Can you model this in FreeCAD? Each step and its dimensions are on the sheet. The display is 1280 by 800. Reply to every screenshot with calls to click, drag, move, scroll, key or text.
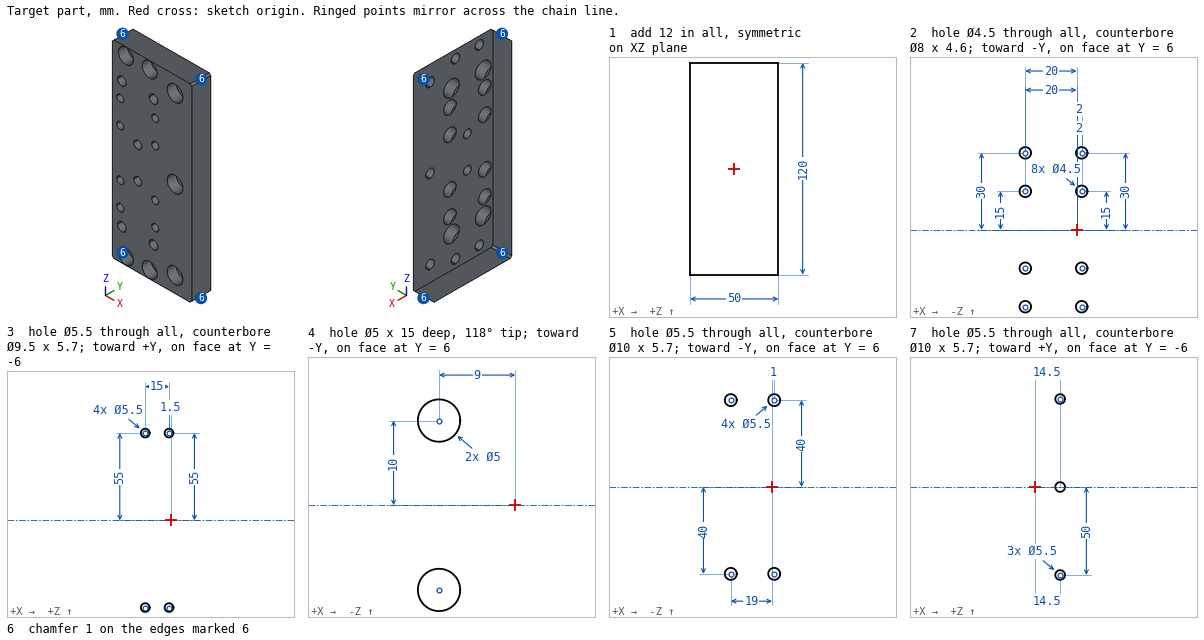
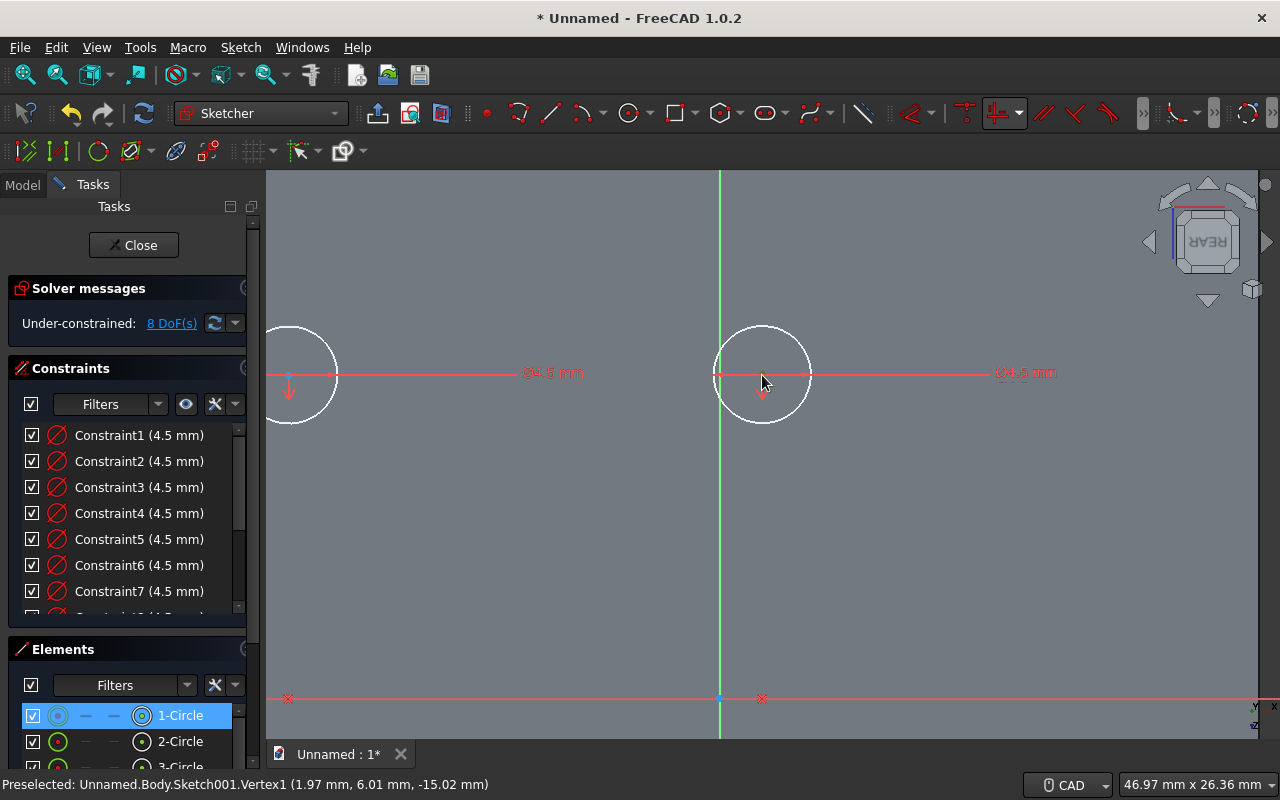
key(l)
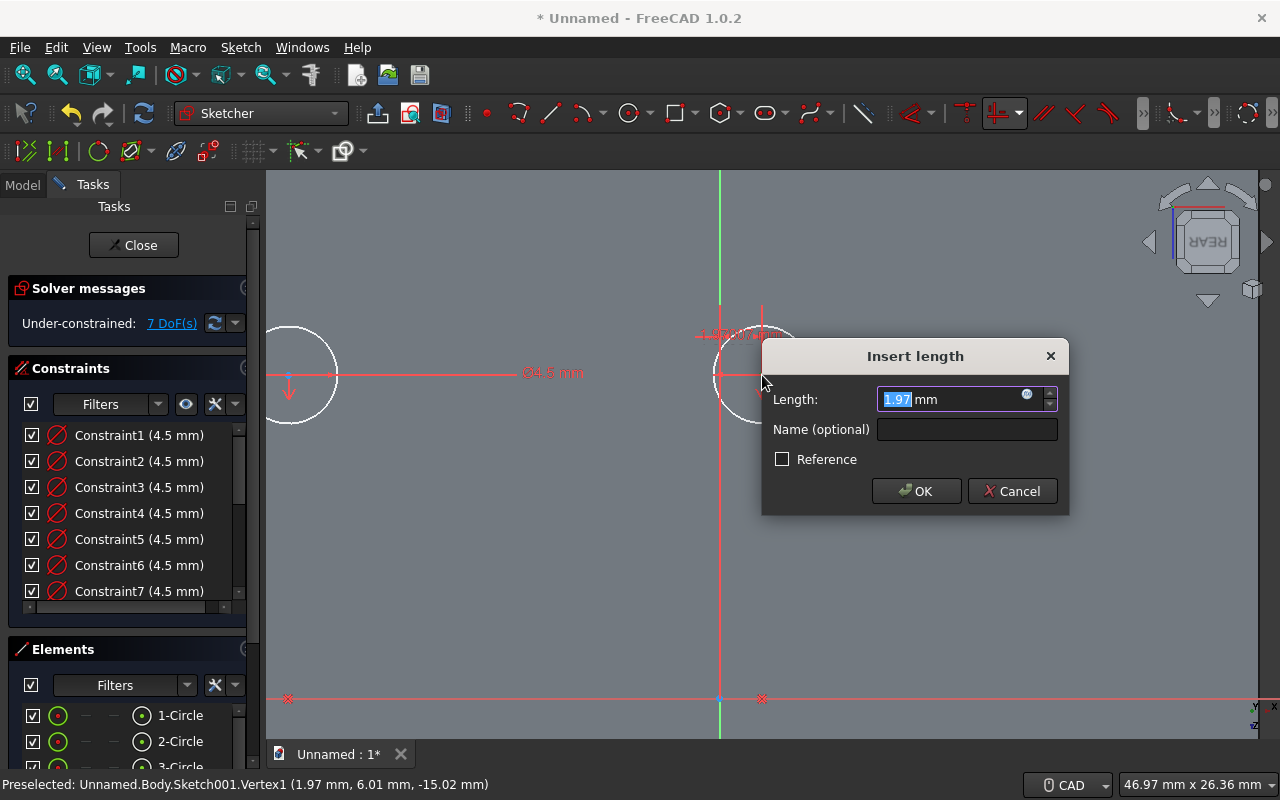
text(2)
key(Return)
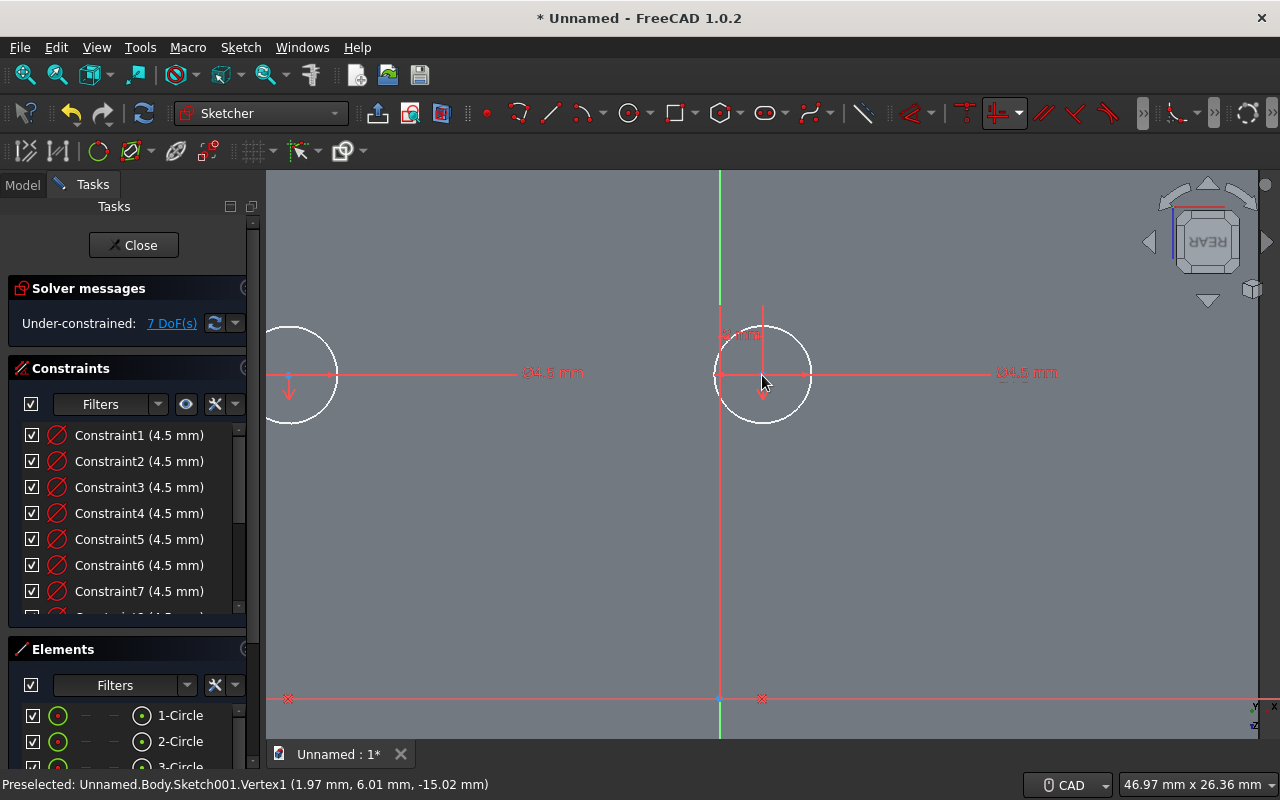
scroll(763, 375, down, 7)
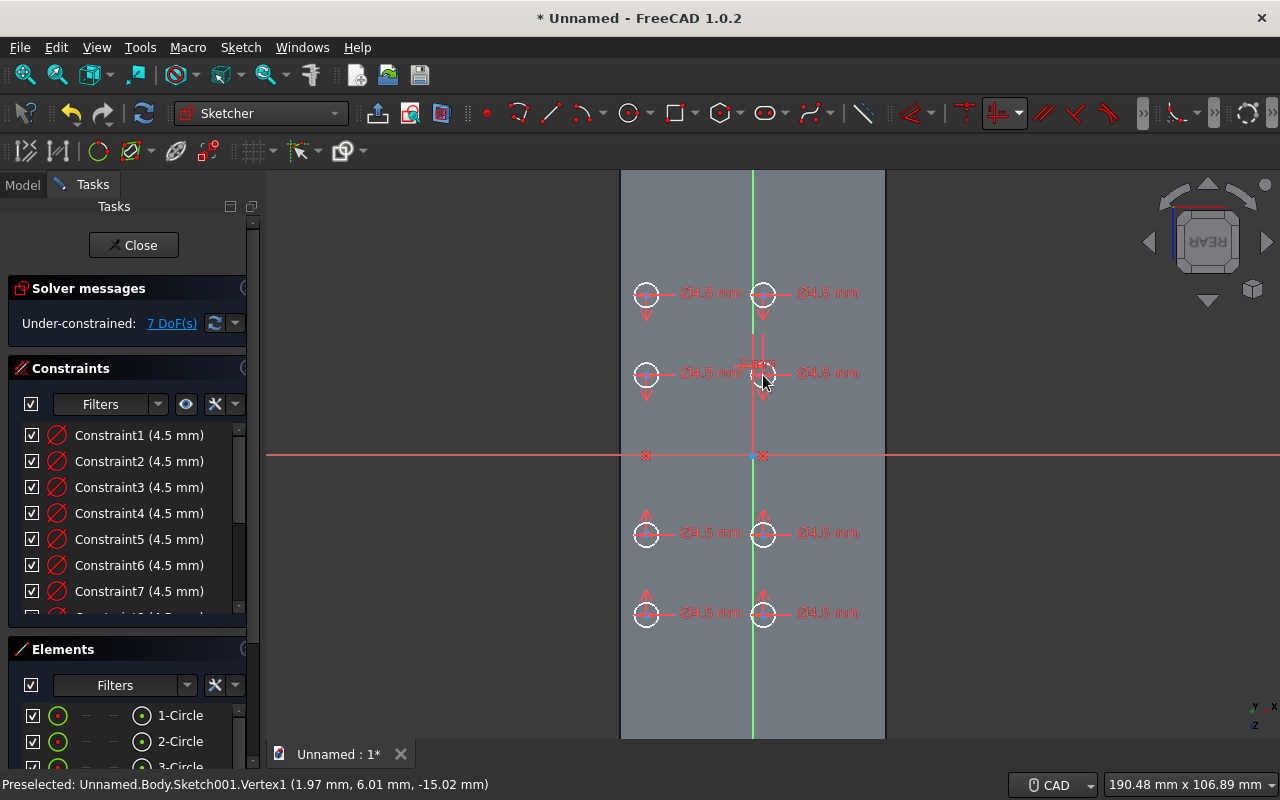
scroll(763, 295, up, 7)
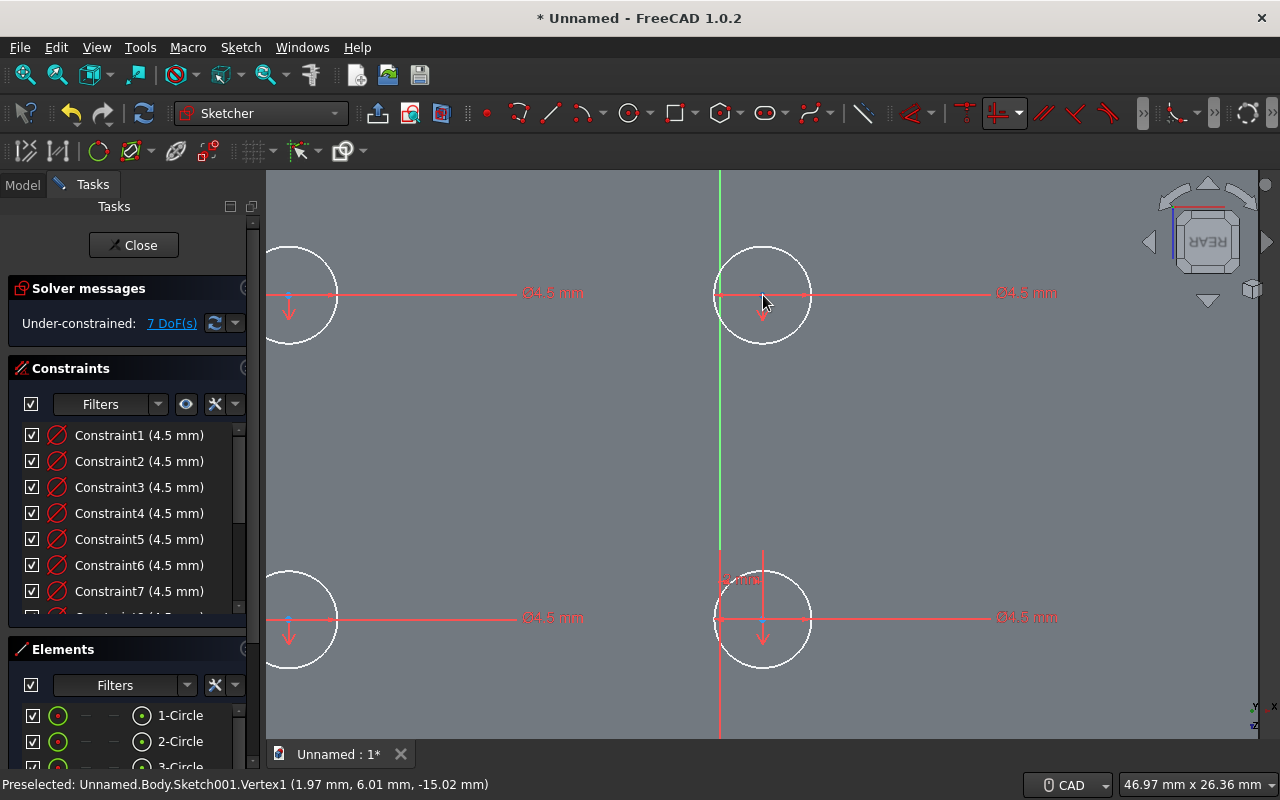
click(763, 295)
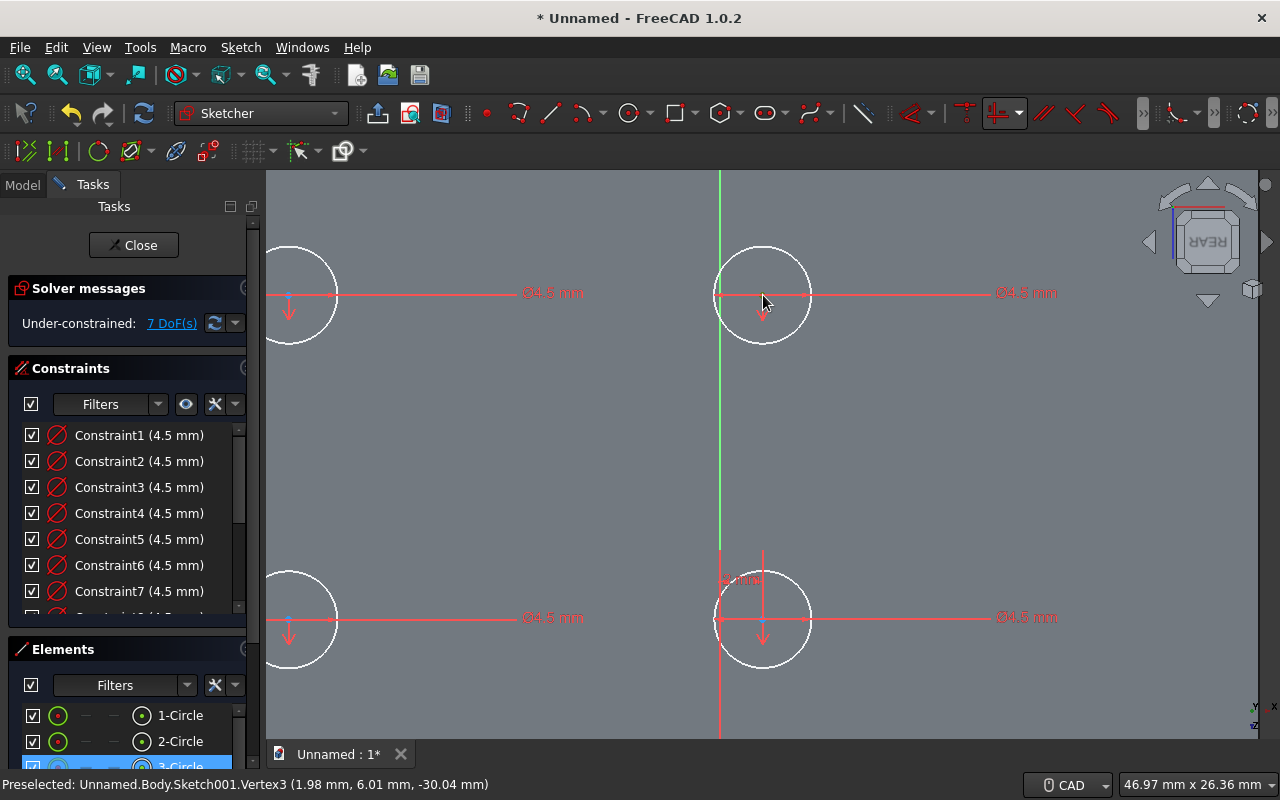
key(l)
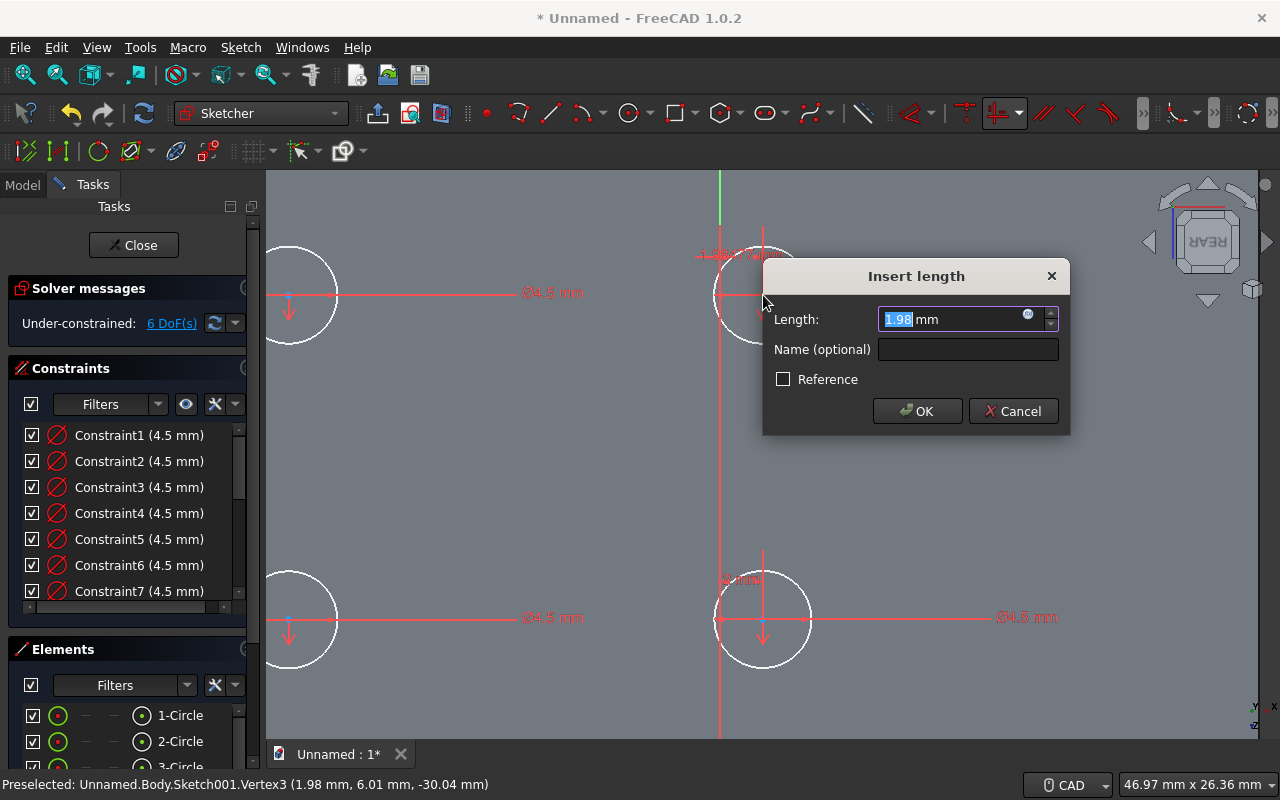
text(2)
key(Return)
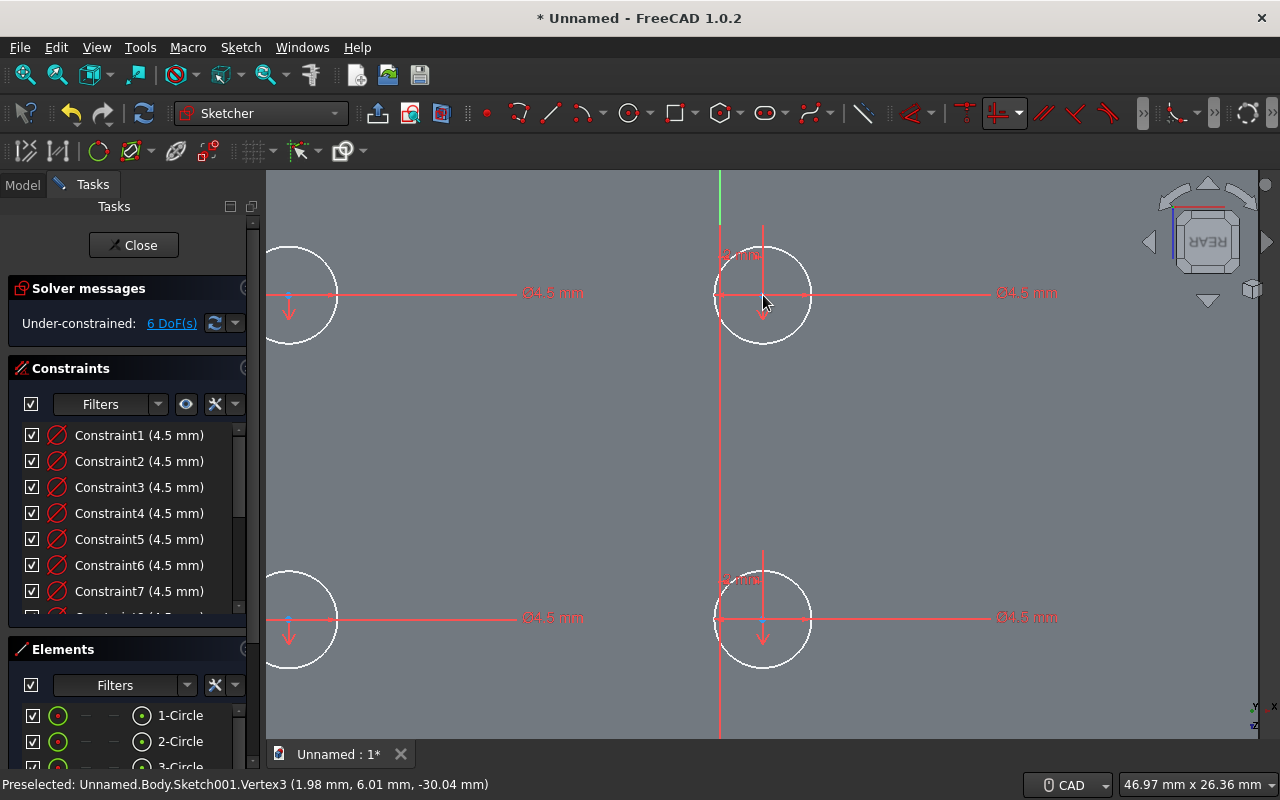
scroll(763, 294, down, 7)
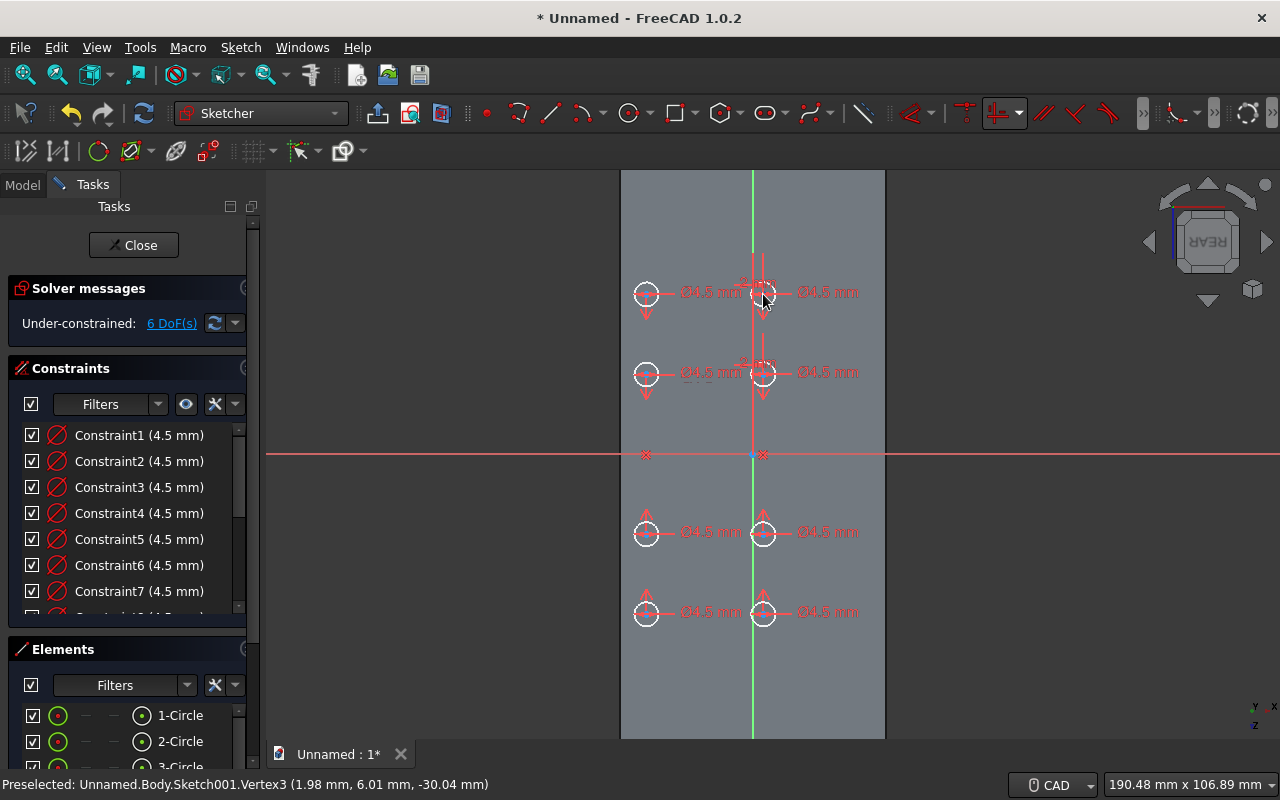
click(763, 374)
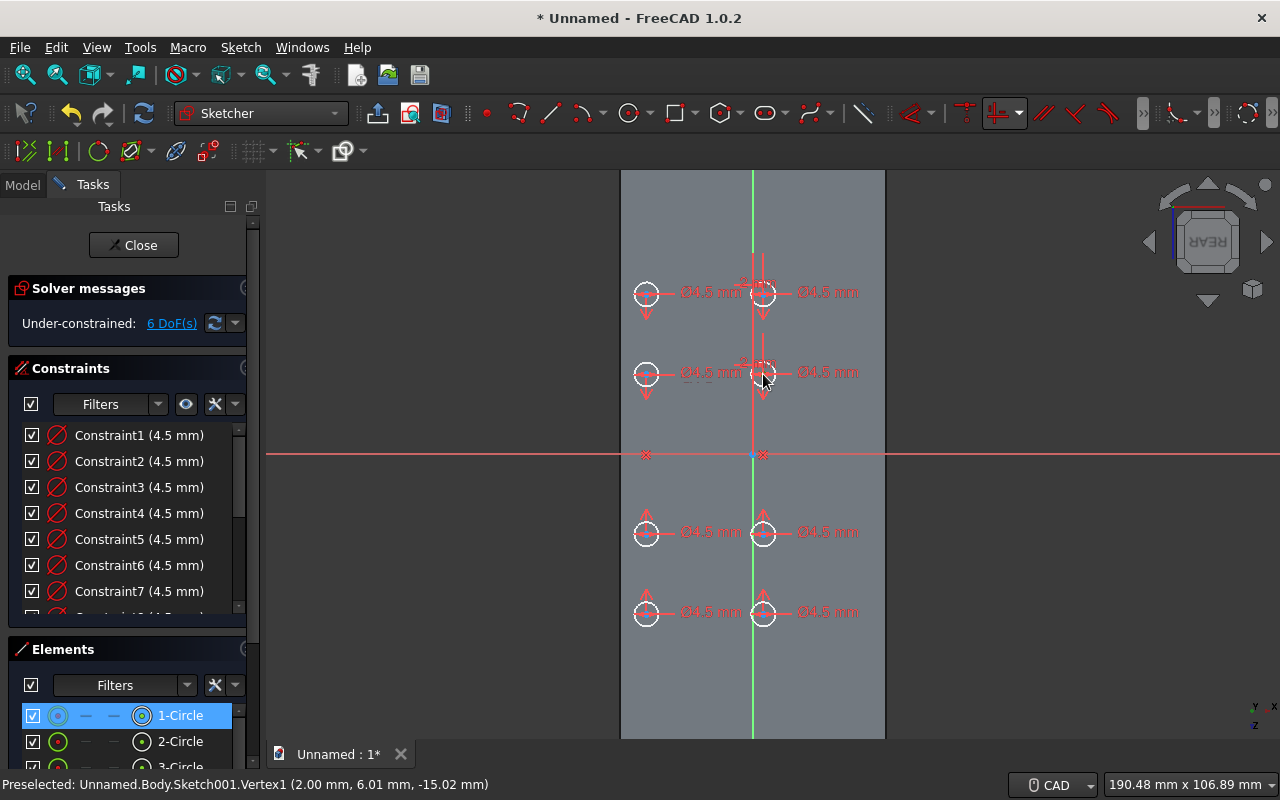
click(934, 114)